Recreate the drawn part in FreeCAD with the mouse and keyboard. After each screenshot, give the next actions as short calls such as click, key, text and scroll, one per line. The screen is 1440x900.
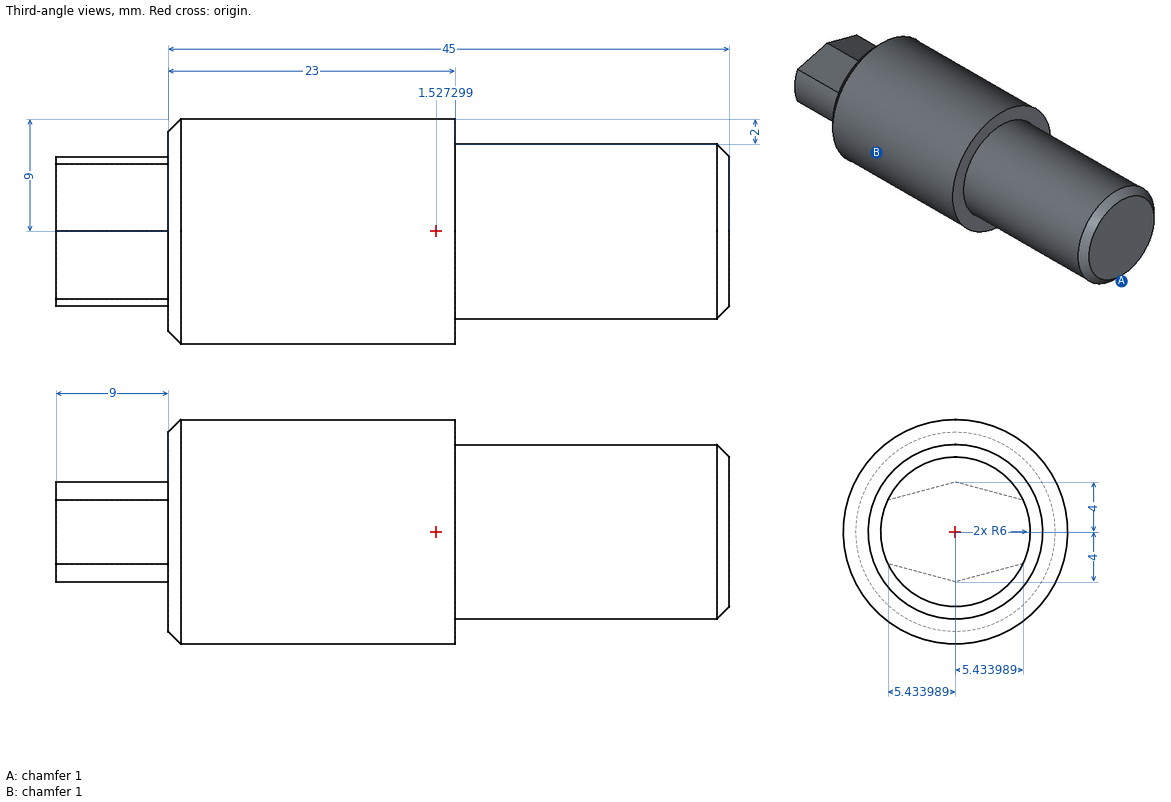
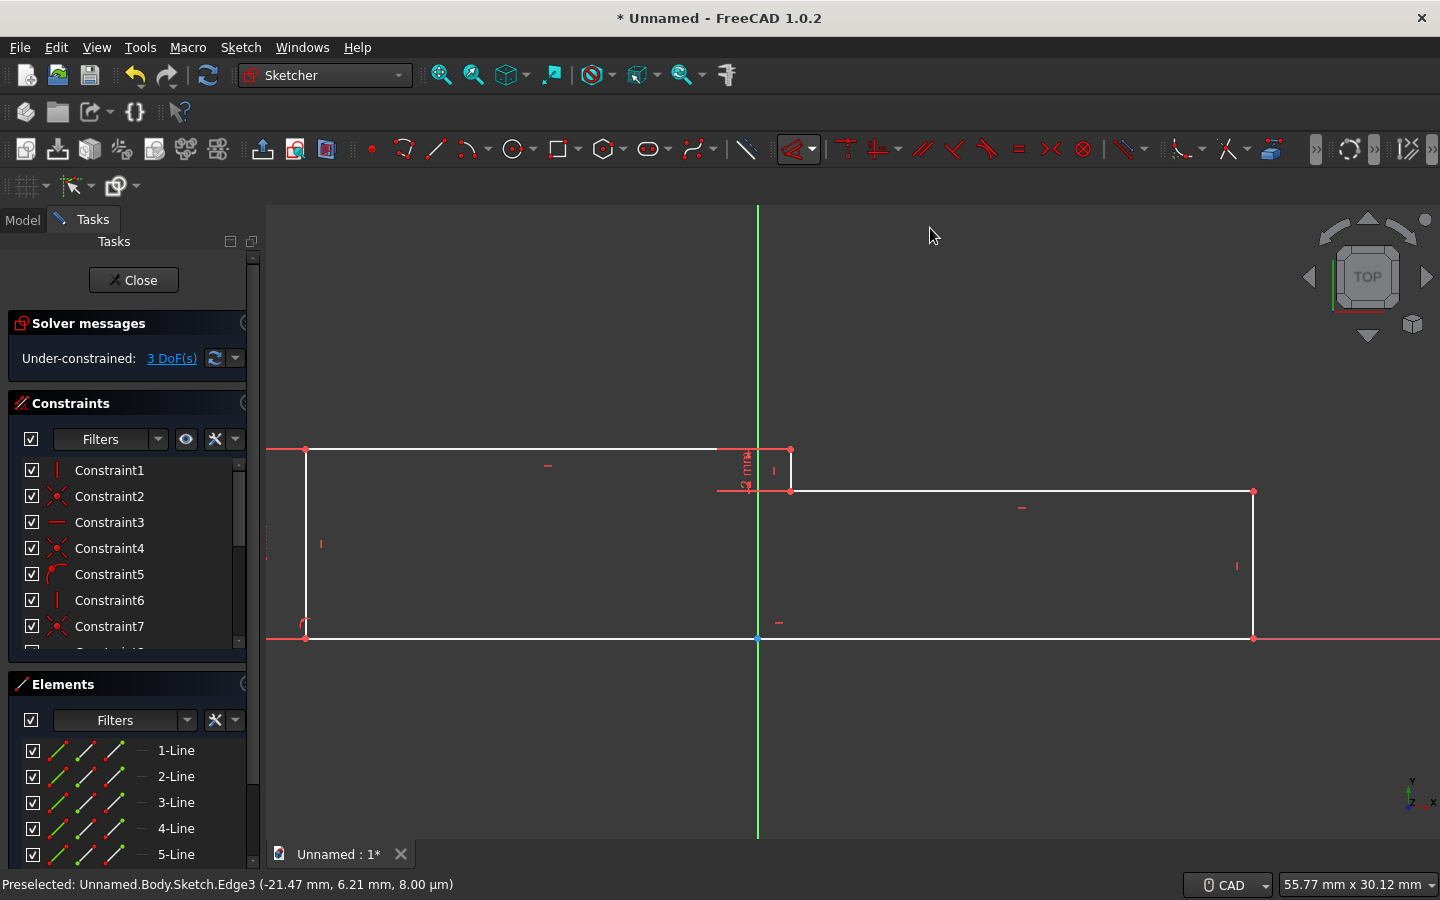
click(645, 449)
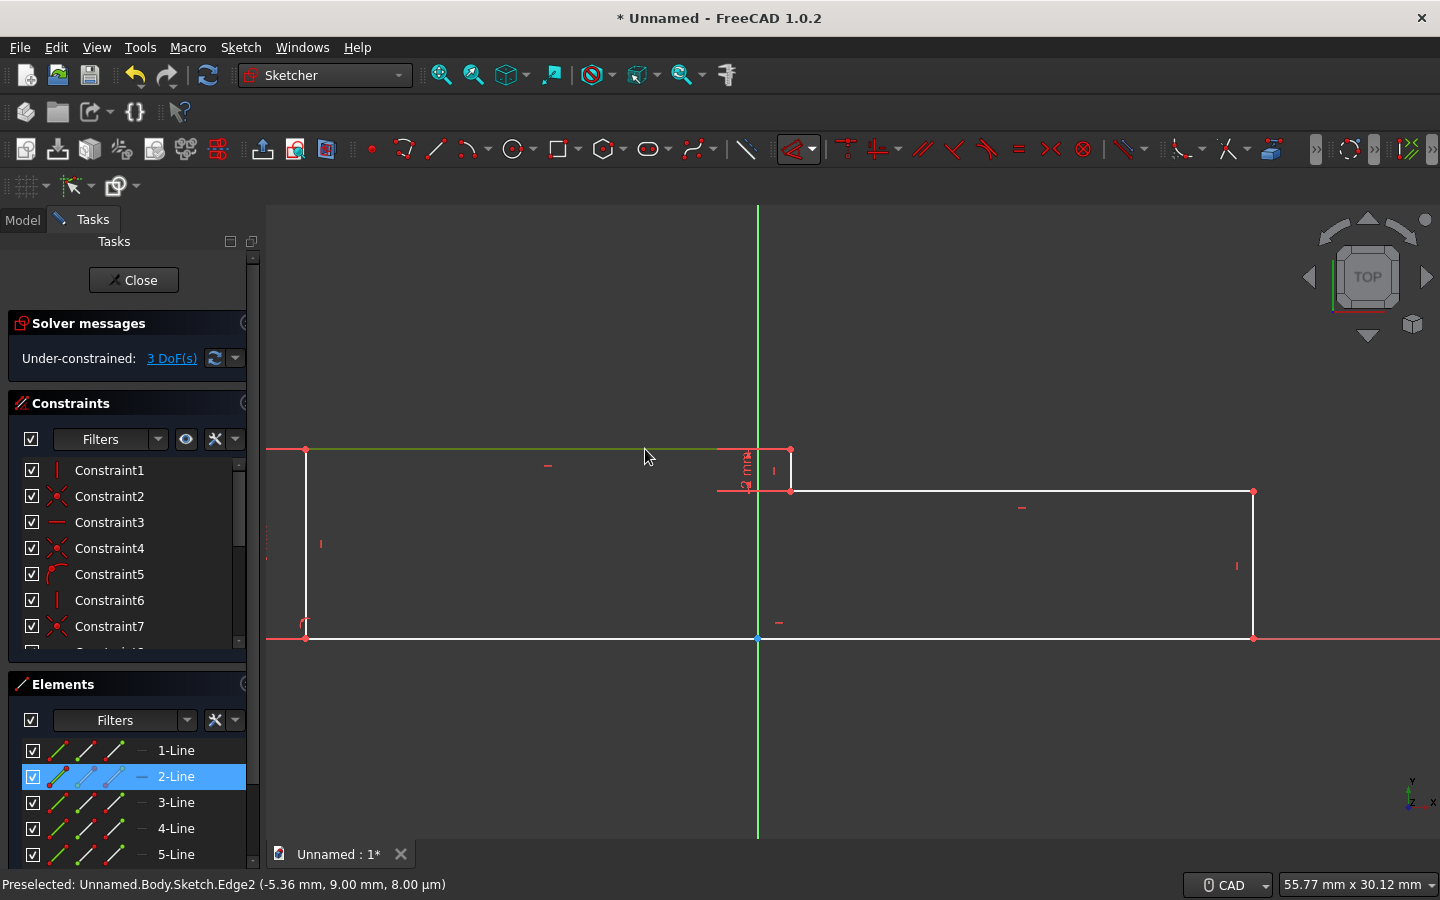
key(l)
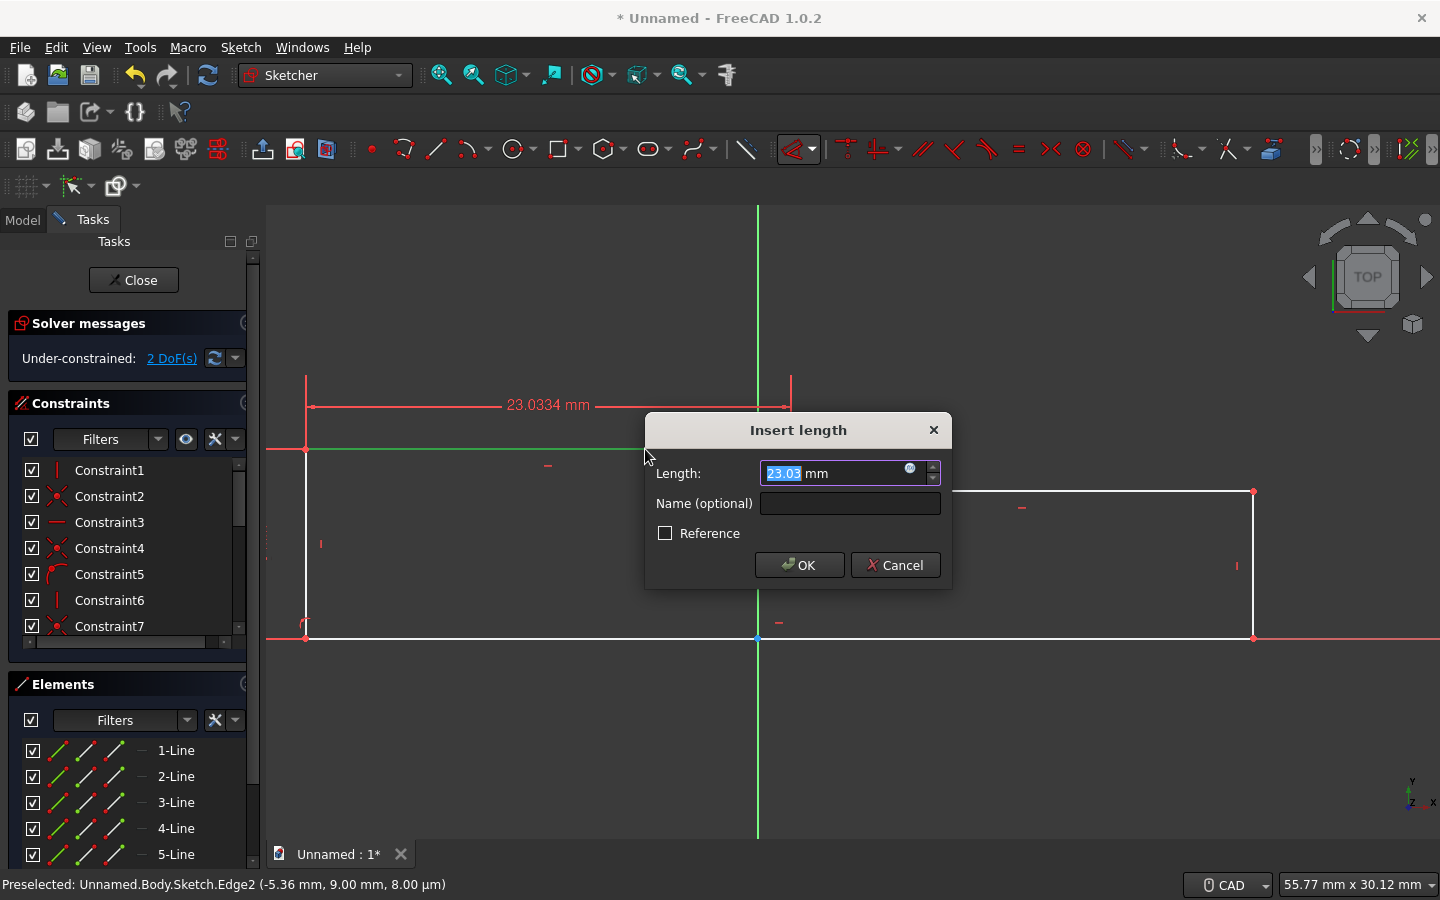
text(23)
key(Return)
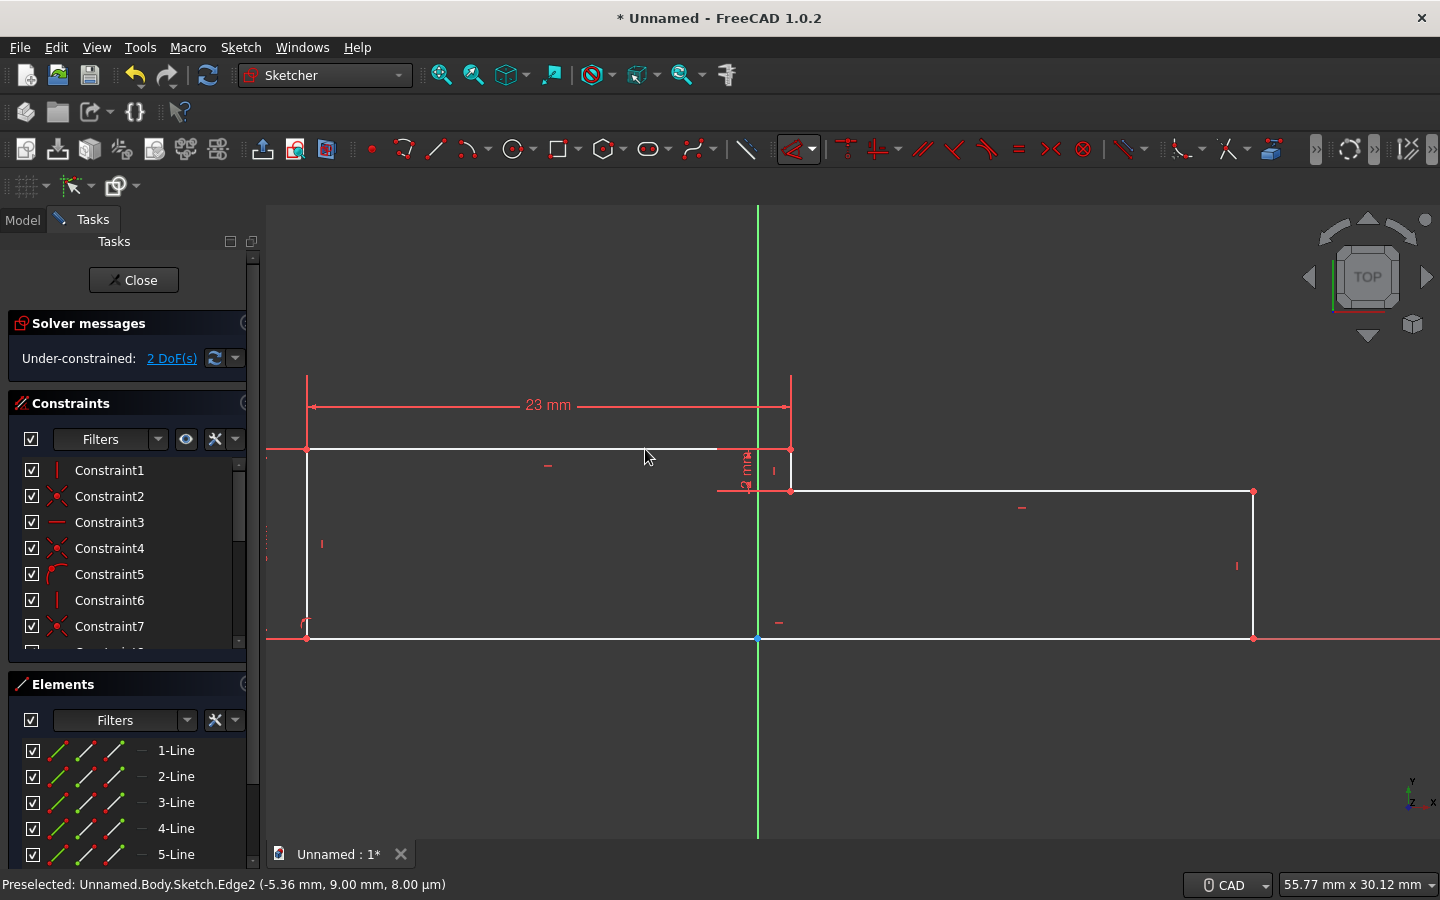
click(591, 639)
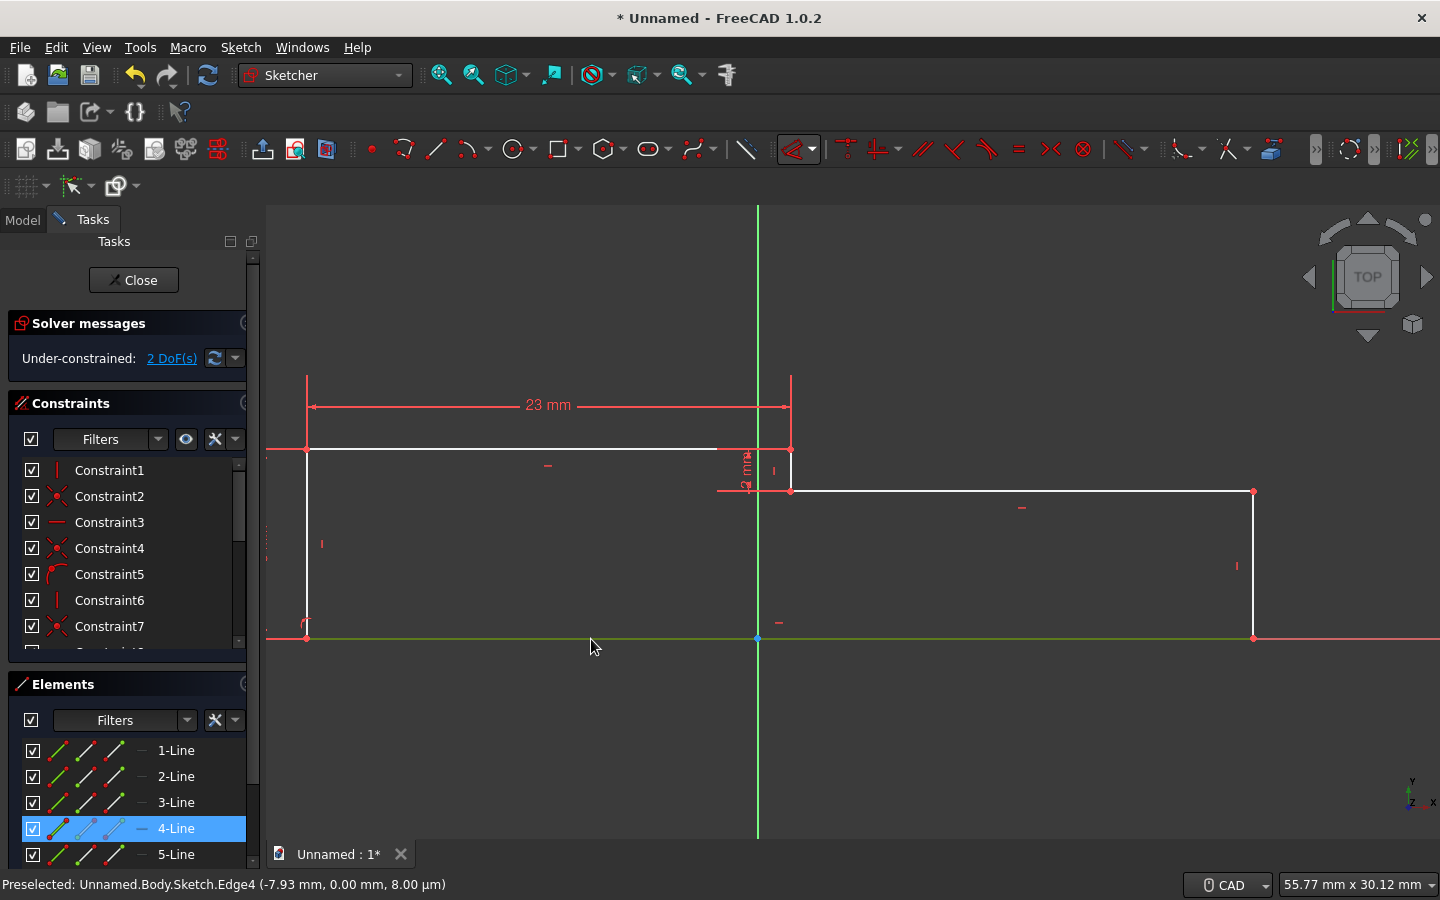
click(814, 150)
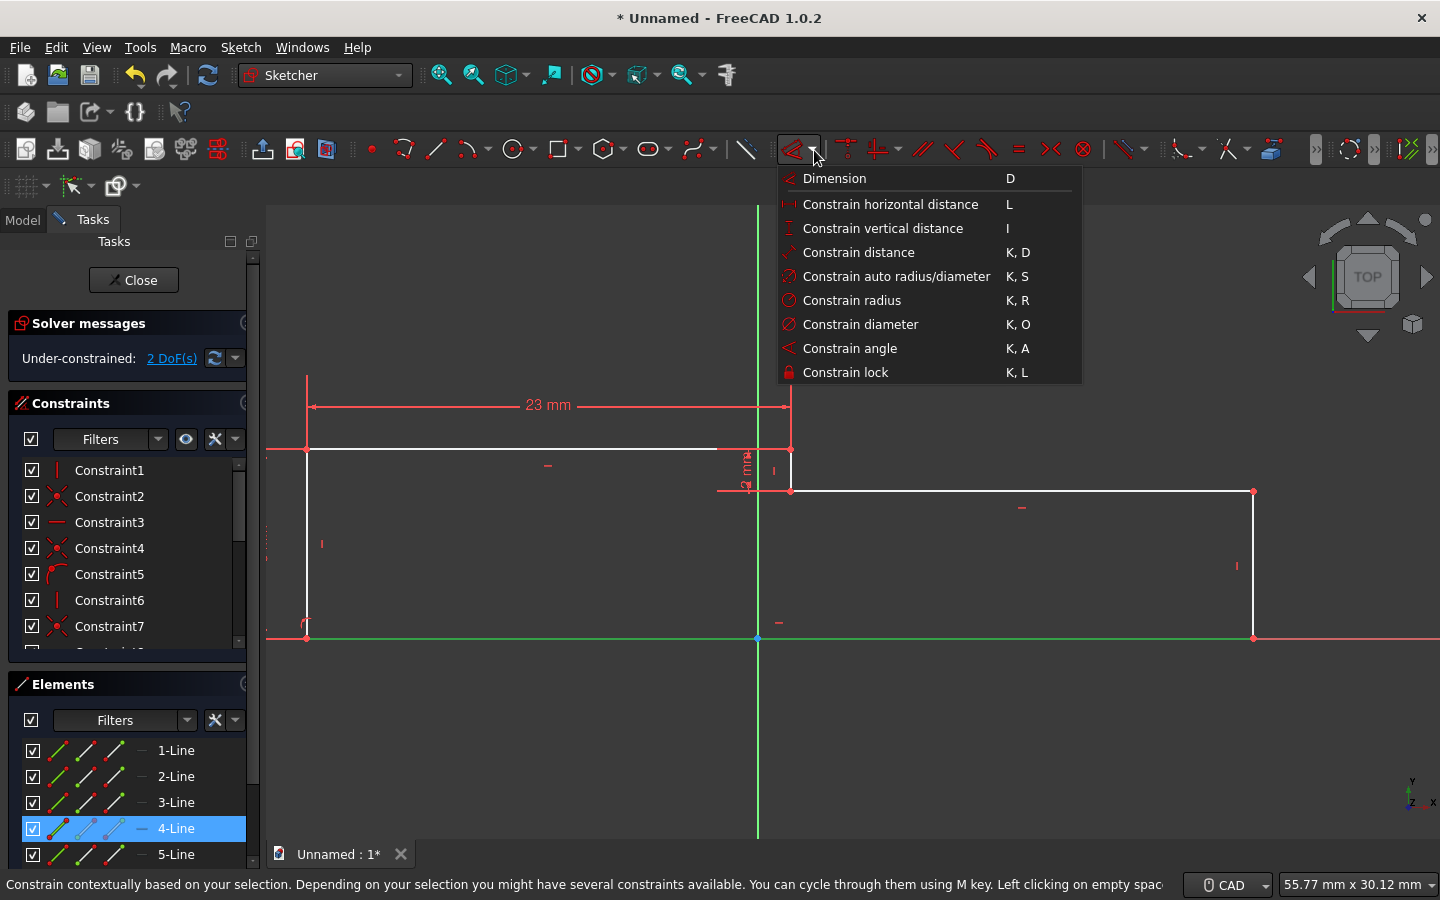
click(930, 204)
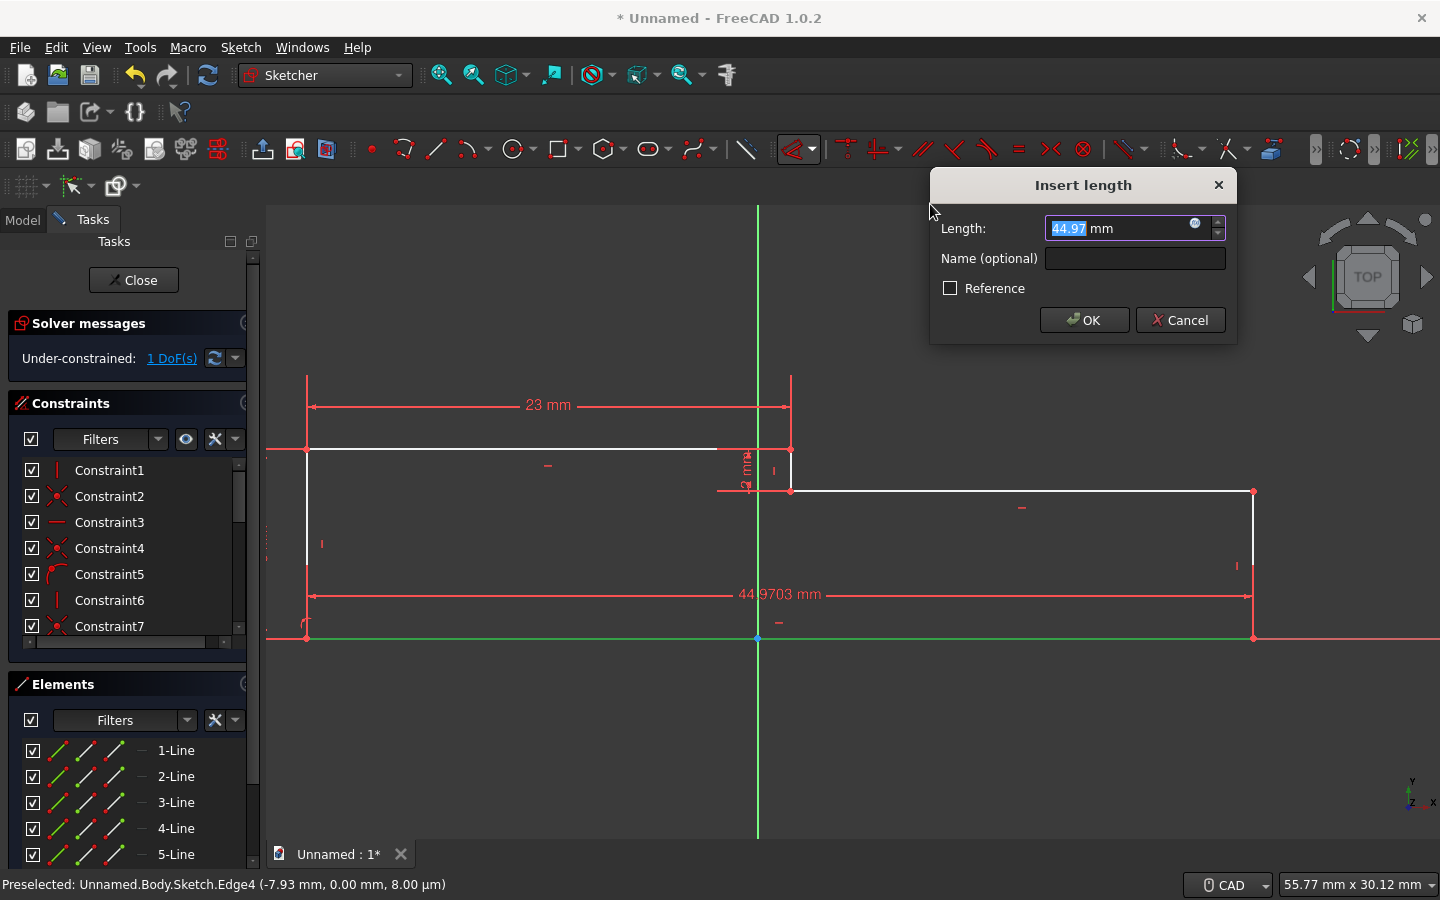
text(45)
key(Return)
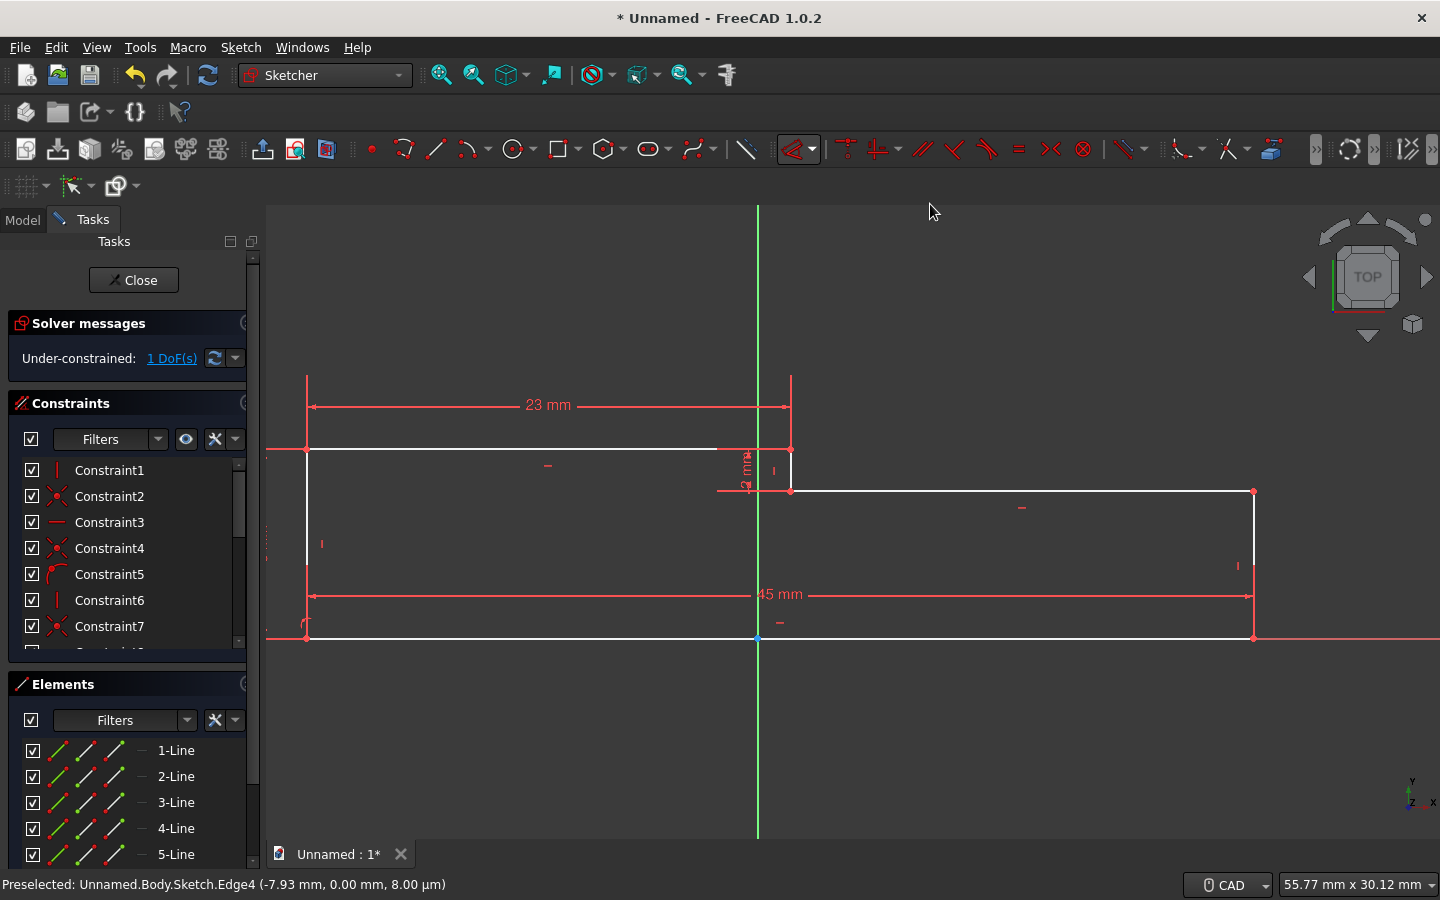
scroll(791, 491, up, 2)